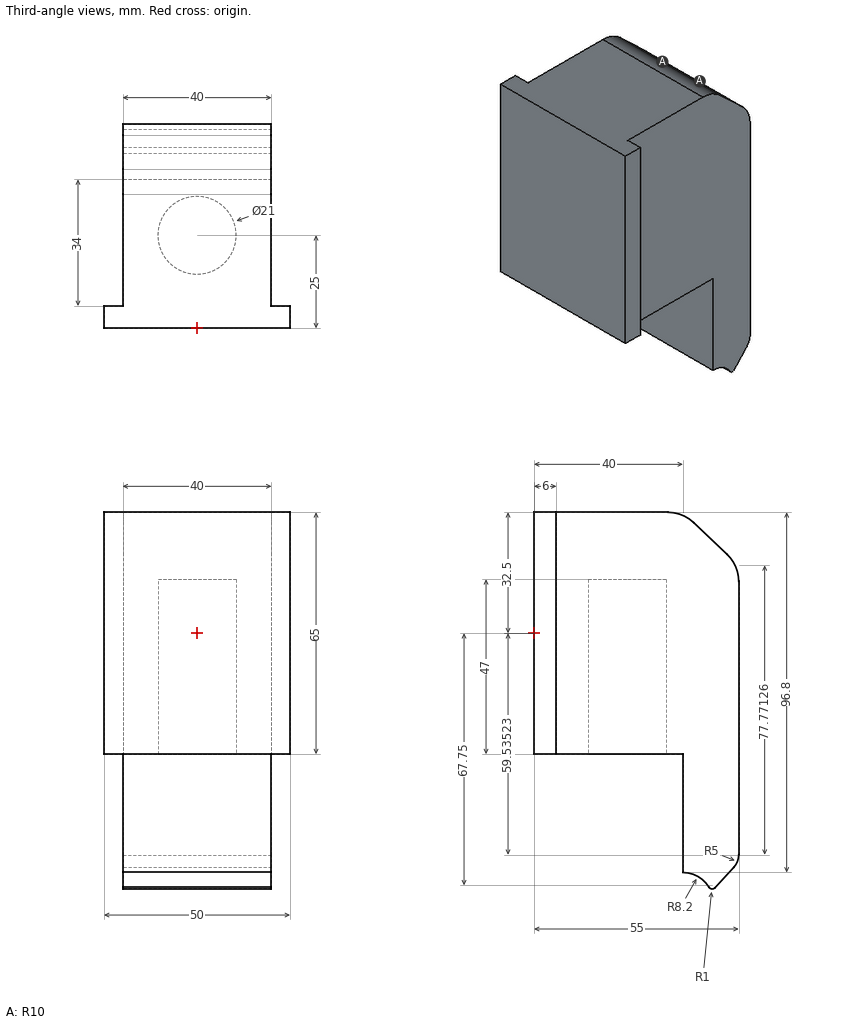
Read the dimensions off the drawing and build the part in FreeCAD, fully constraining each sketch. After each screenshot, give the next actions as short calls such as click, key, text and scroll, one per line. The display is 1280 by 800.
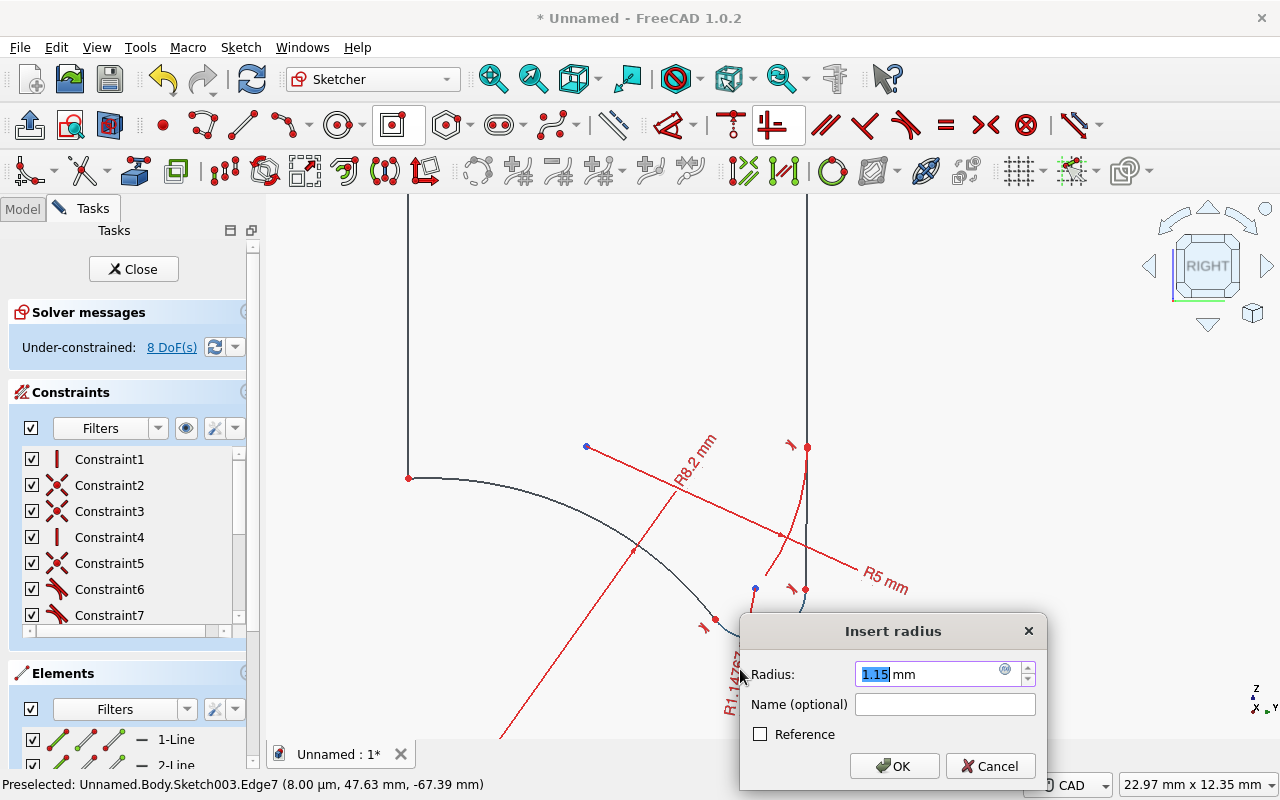
text(1)
key(Return)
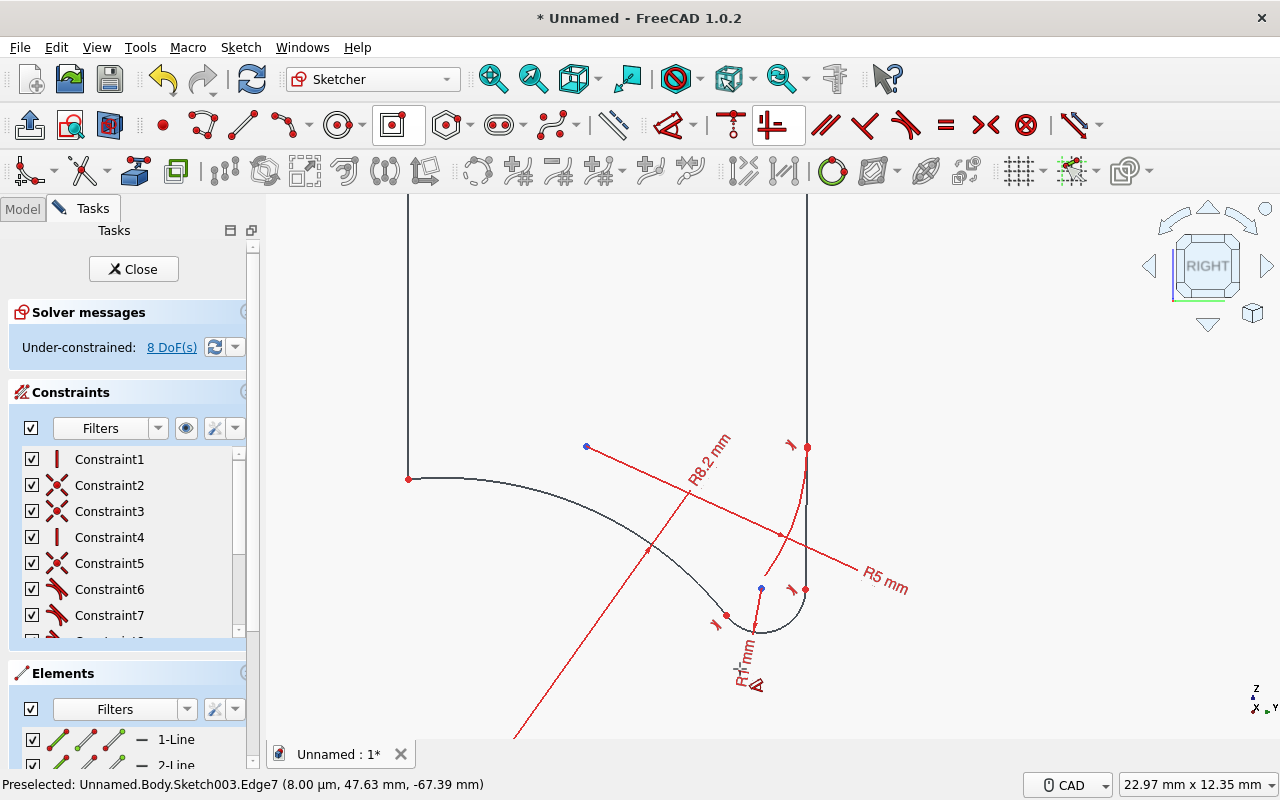
scroll(807, 446, up, 4)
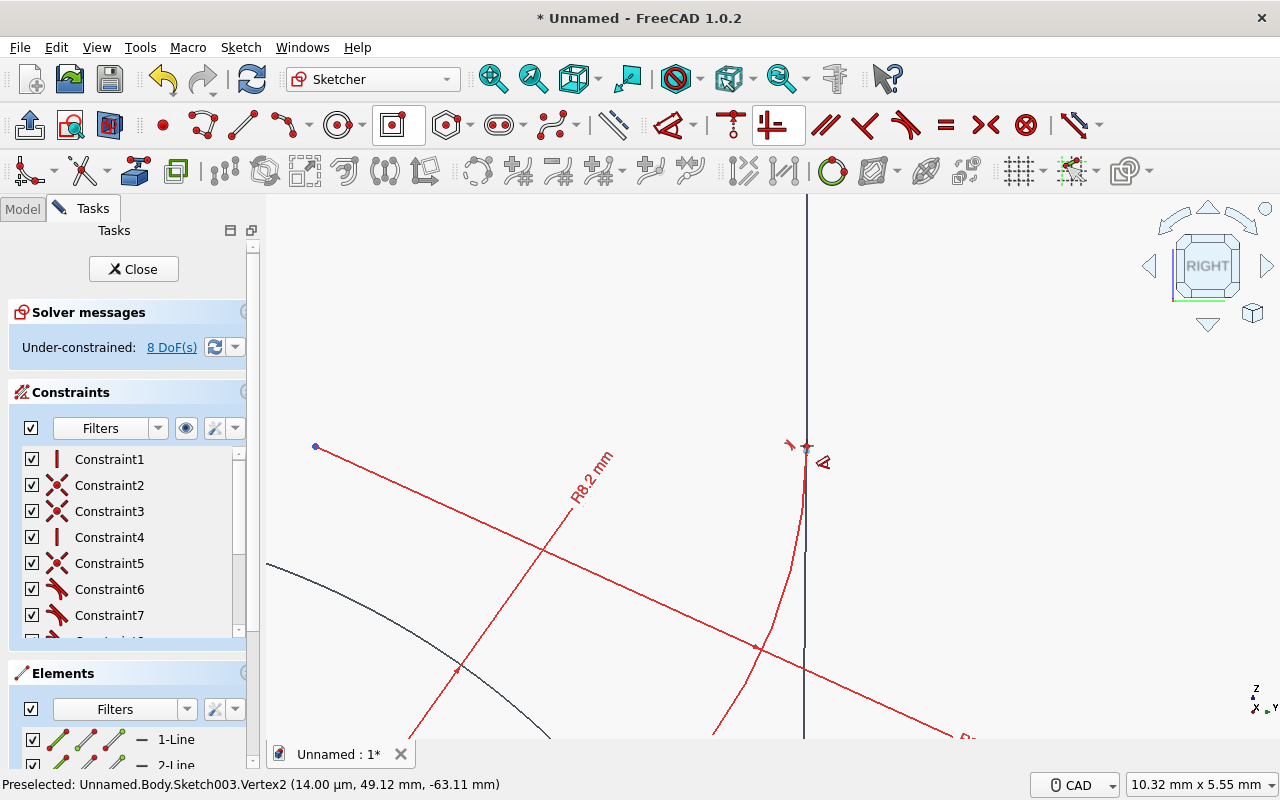
click(805, 444)
click(432, 480)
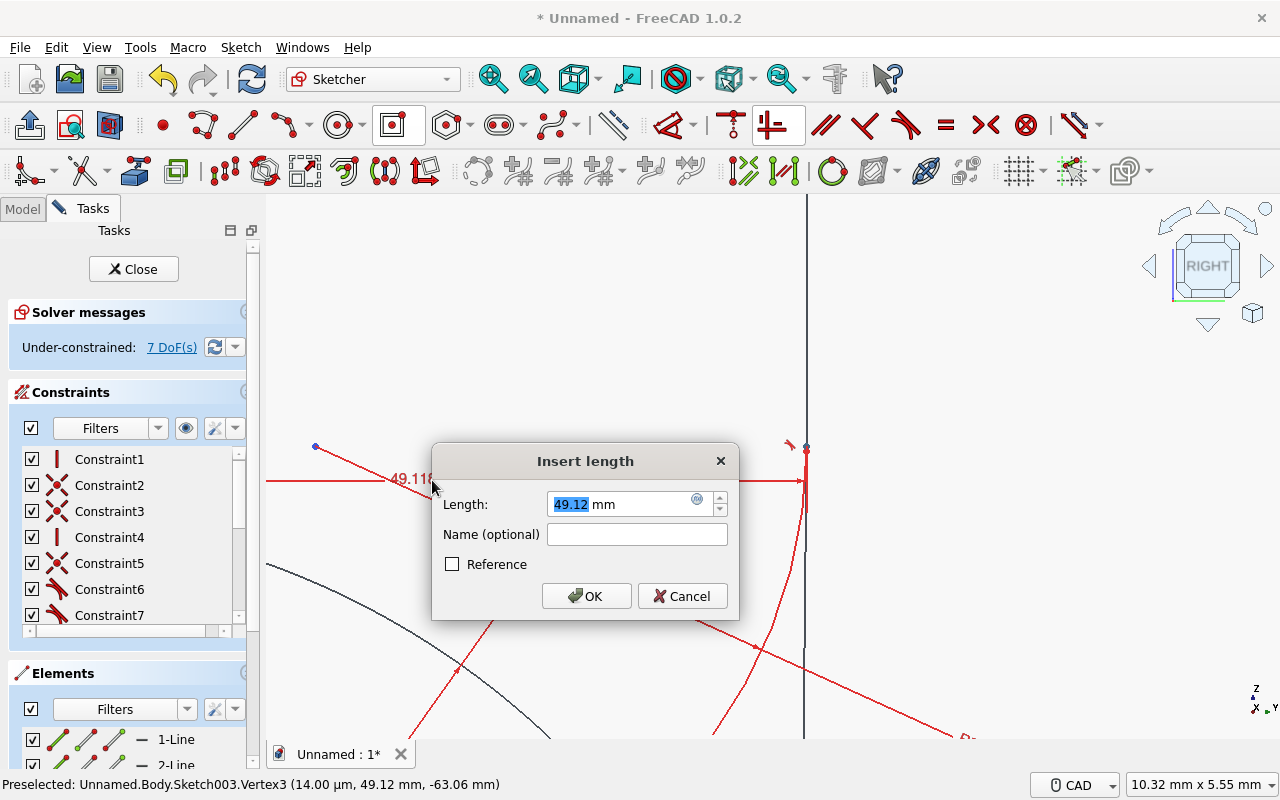
text(55)
key(Return)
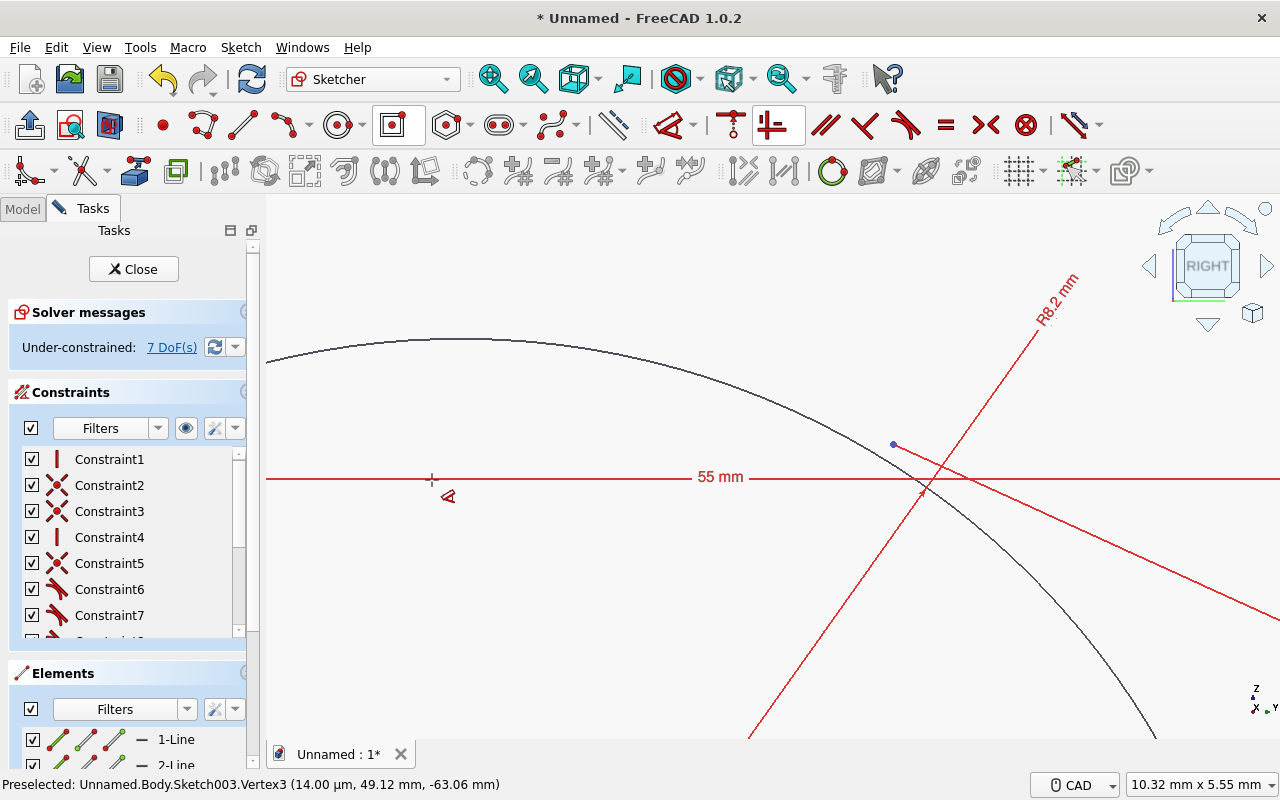
scroll(790, 655, down, 16)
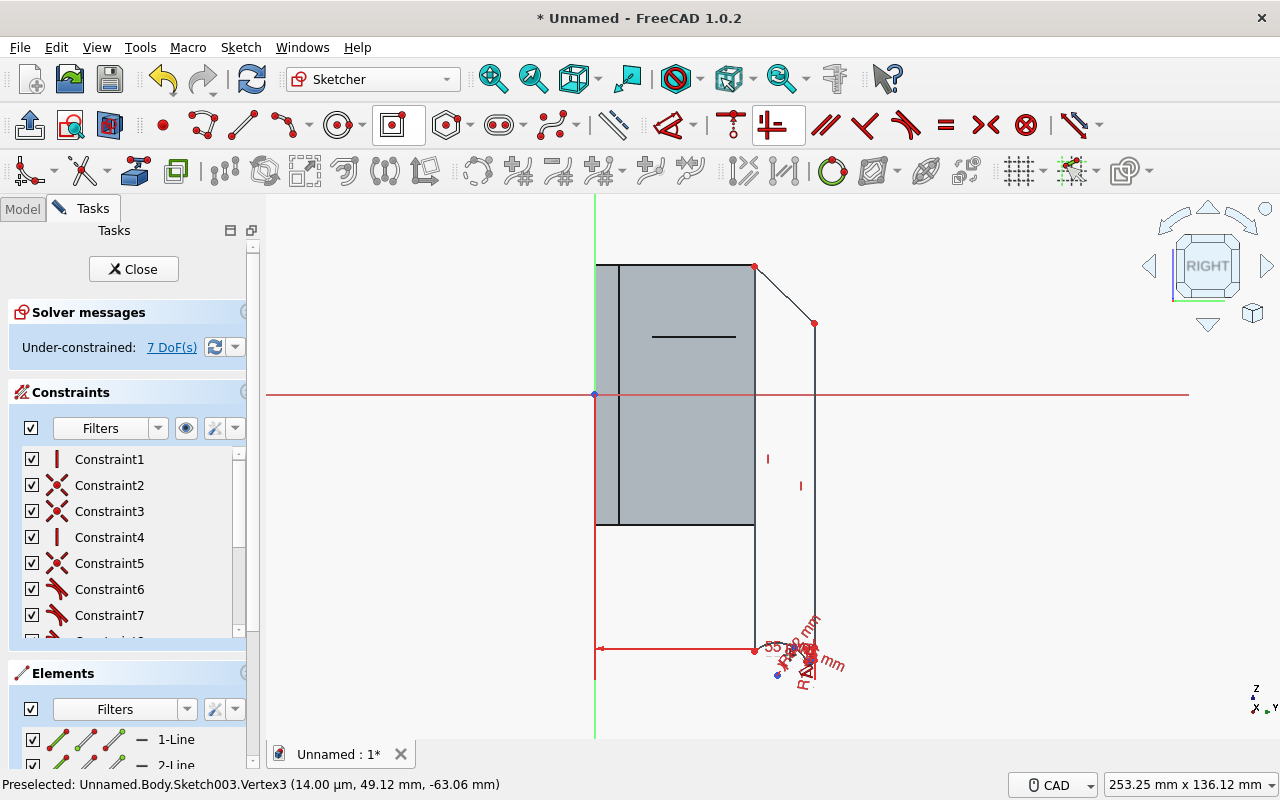
click(755, 266)
click(675, 232)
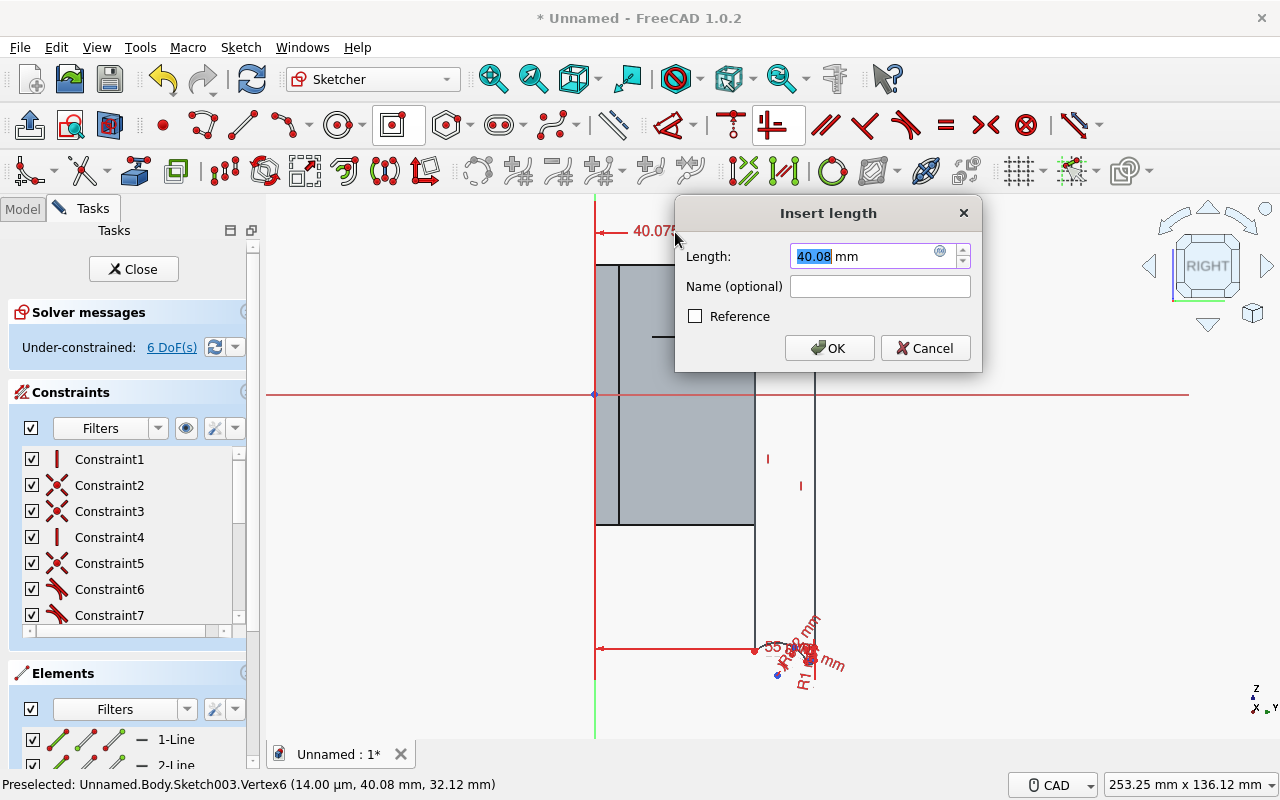
text(40)
key(Return)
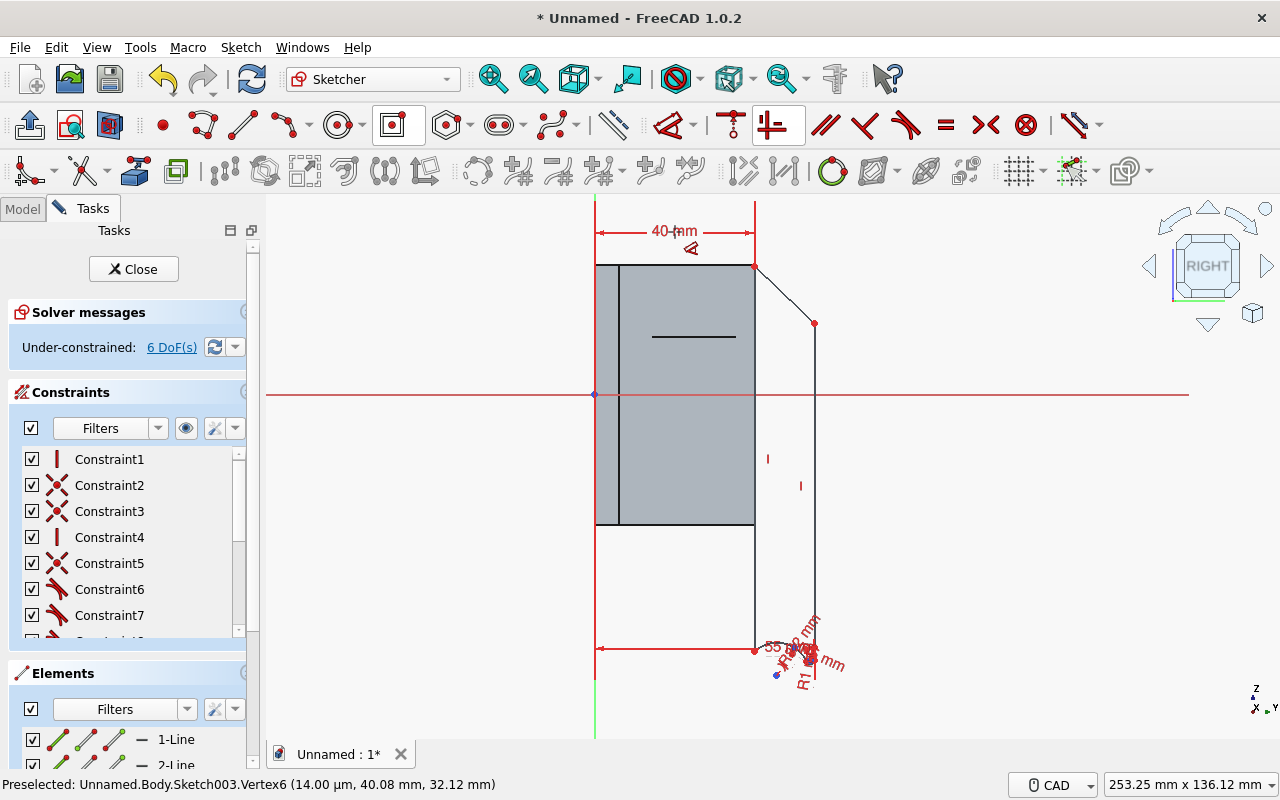
click(777, 676)
click(686, 710)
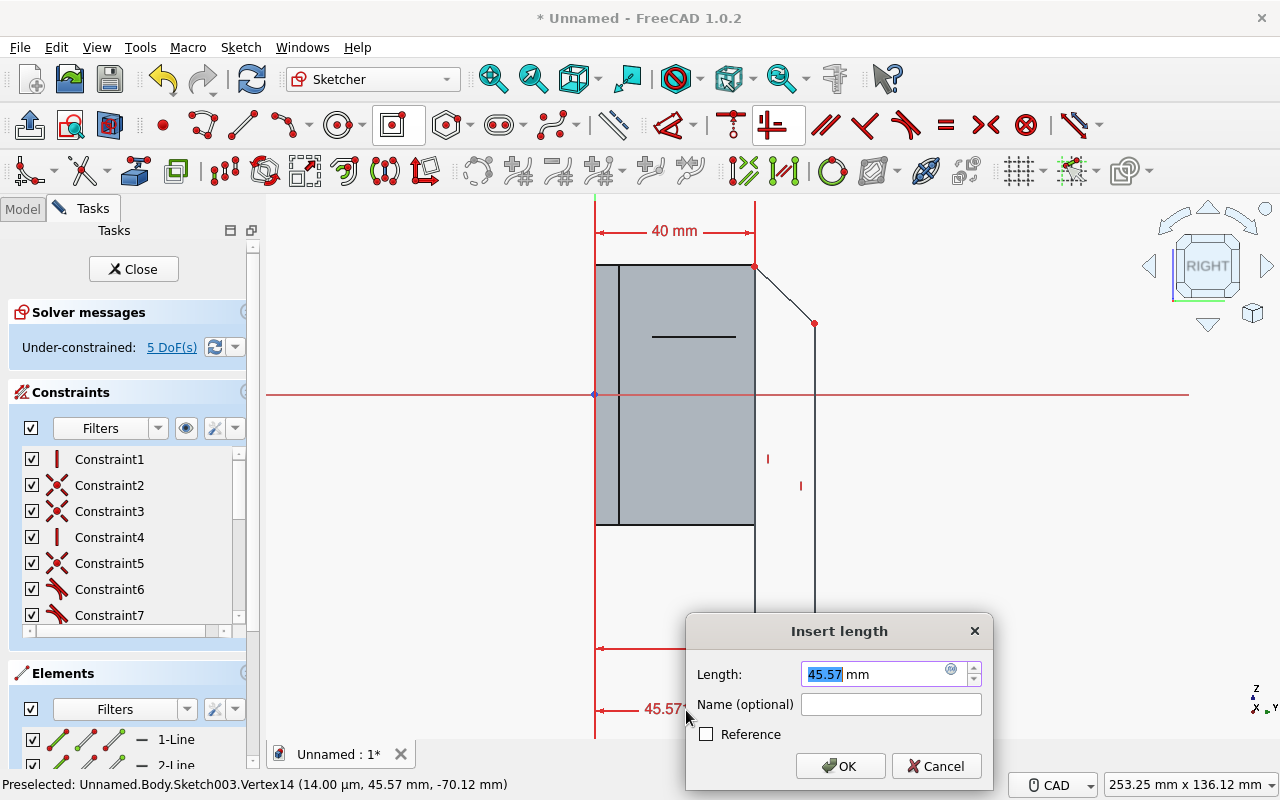
text(40)
key(Return)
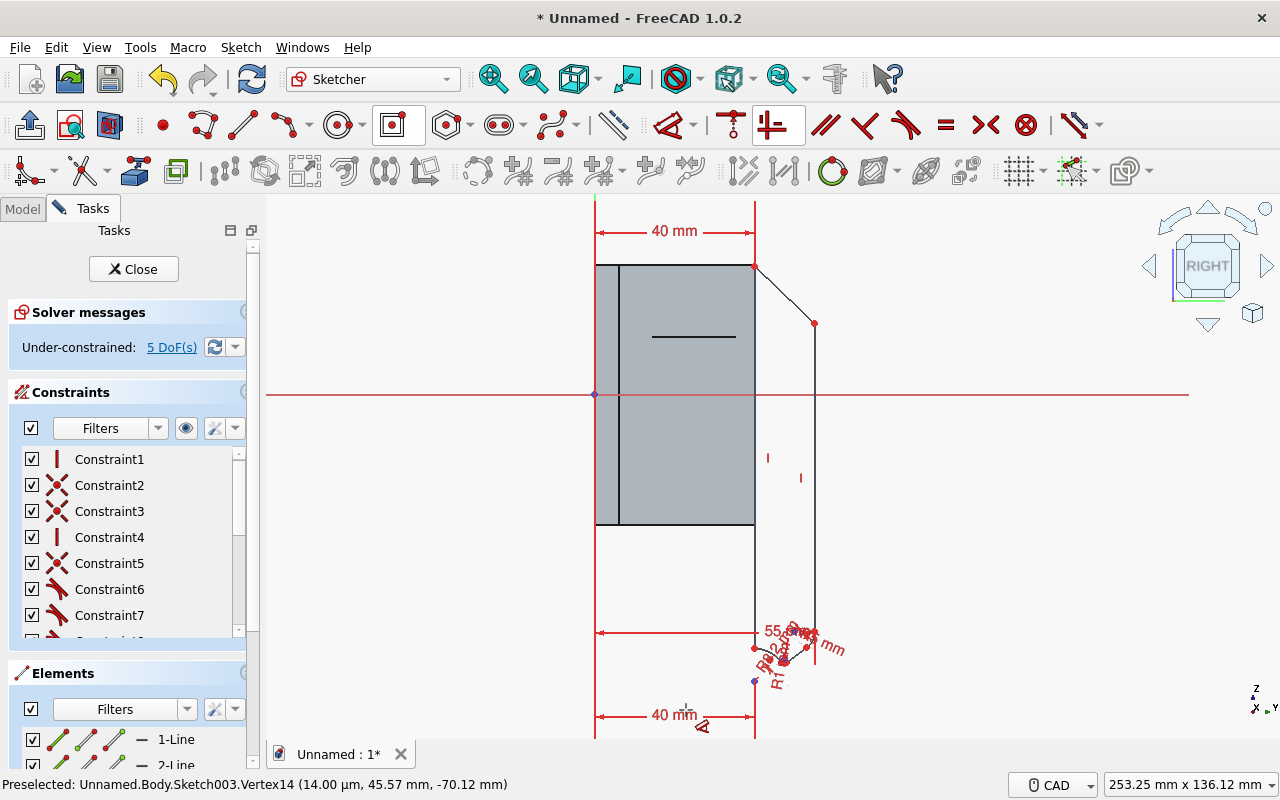
click(755, 381)
click(789, 457)